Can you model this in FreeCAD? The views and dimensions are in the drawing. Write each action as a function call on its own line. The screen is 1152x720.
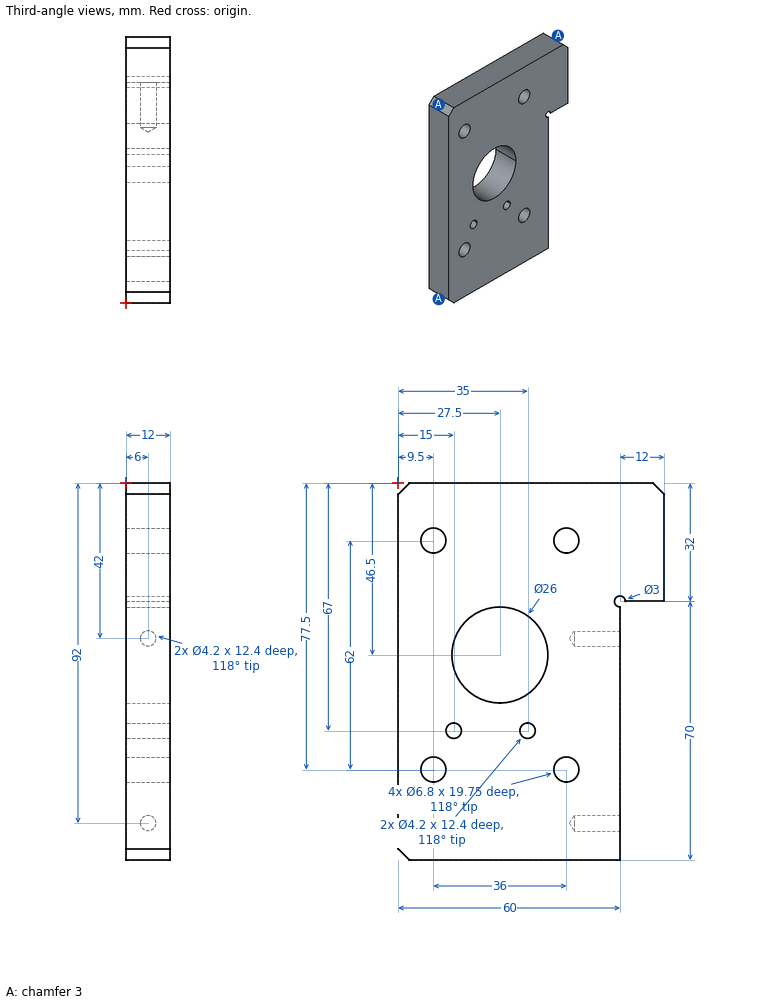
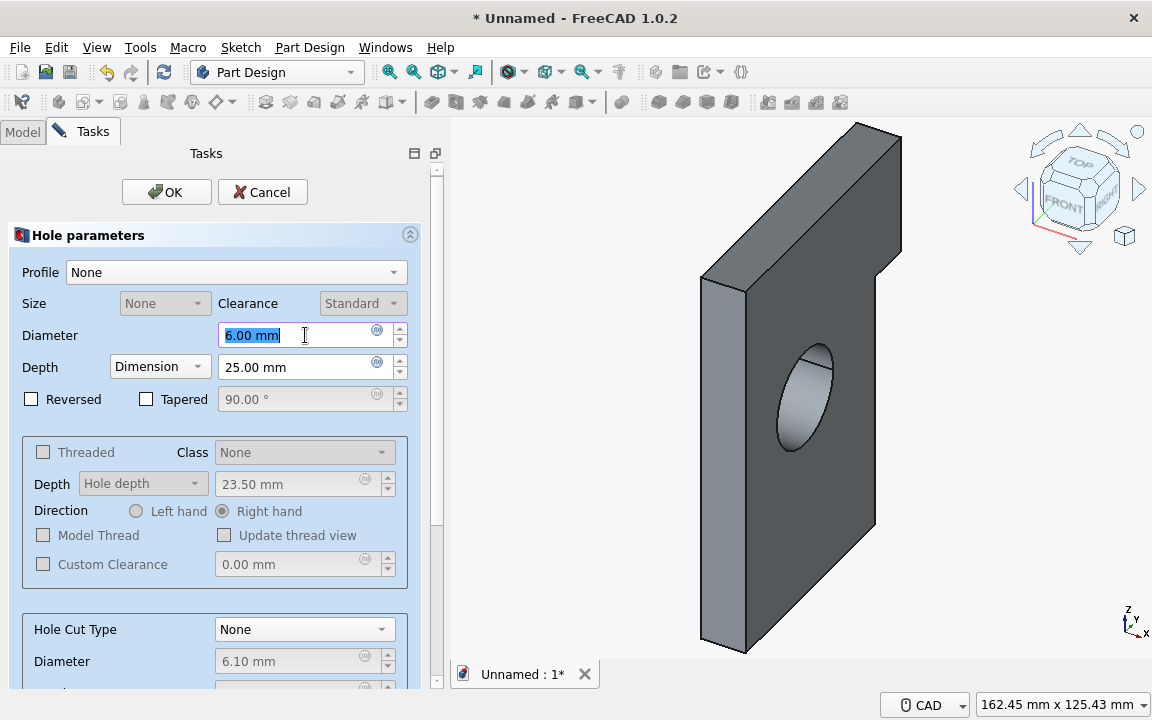
text(6.8)
key(Tab)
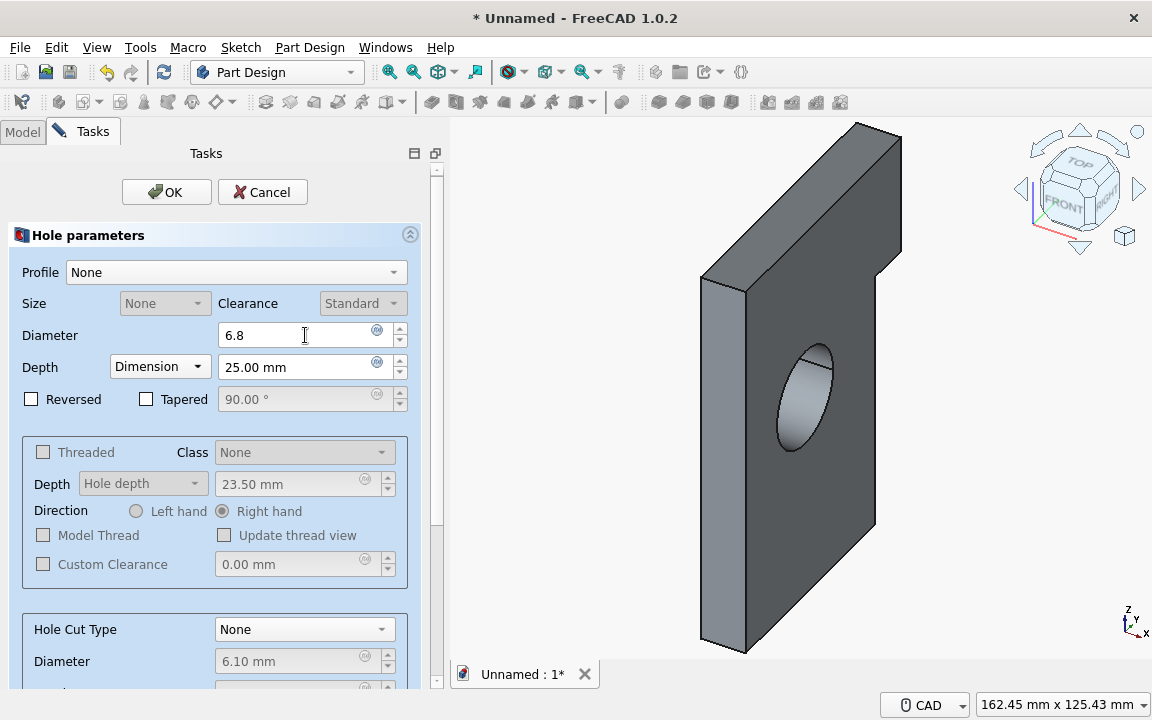
triple_click(305, 367)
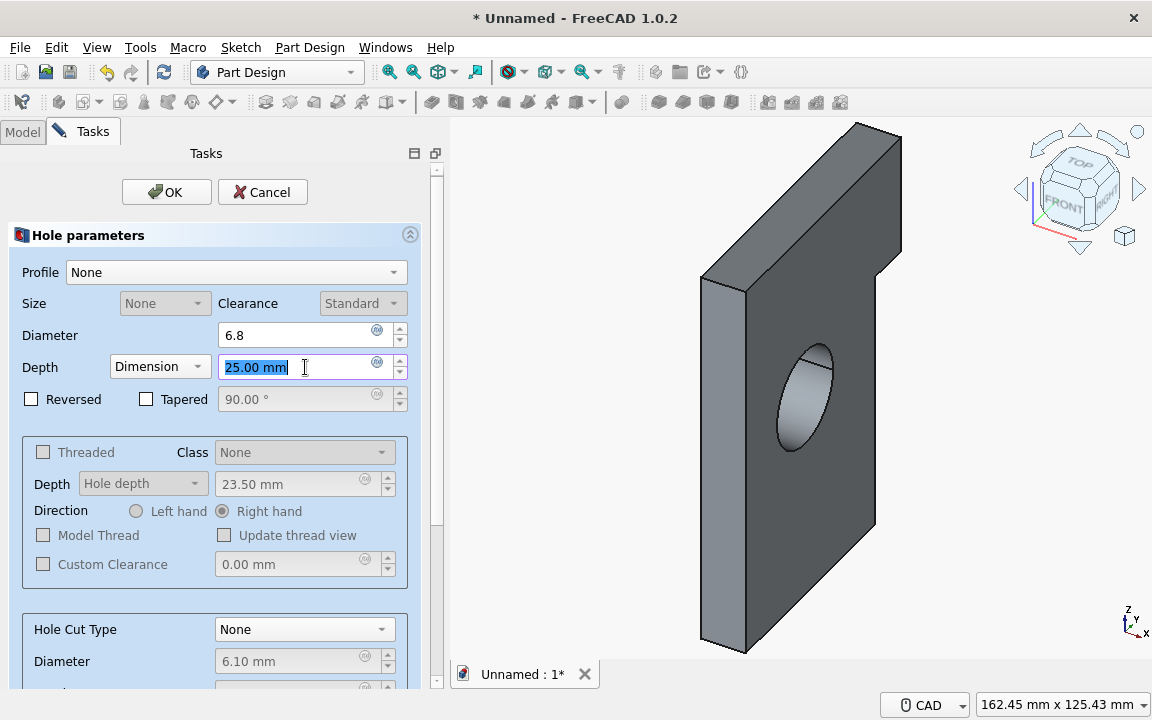
text(19.75)
key(Tab)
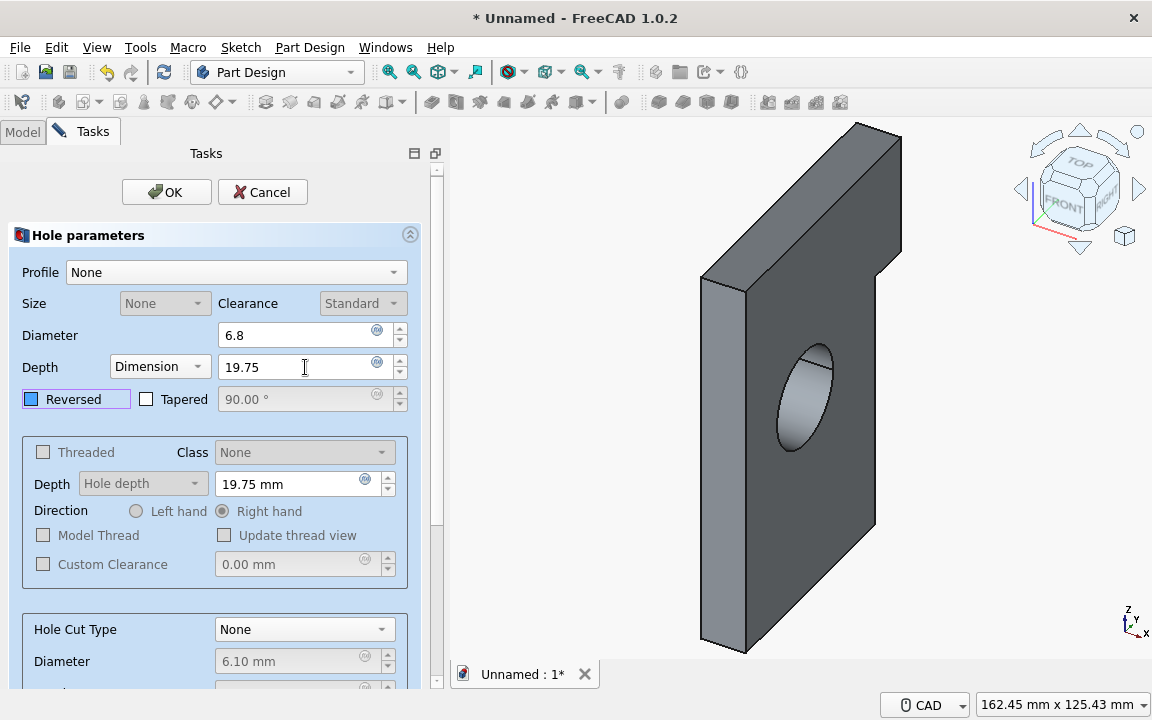
click(30, 399)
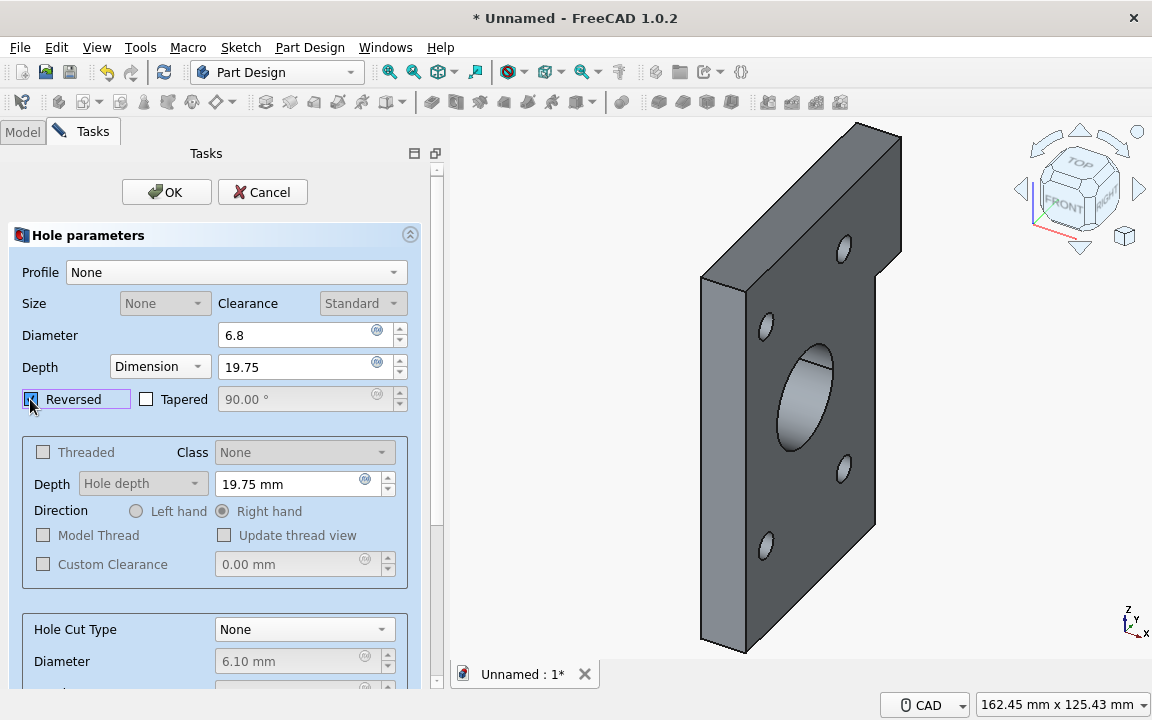
click(167, 192)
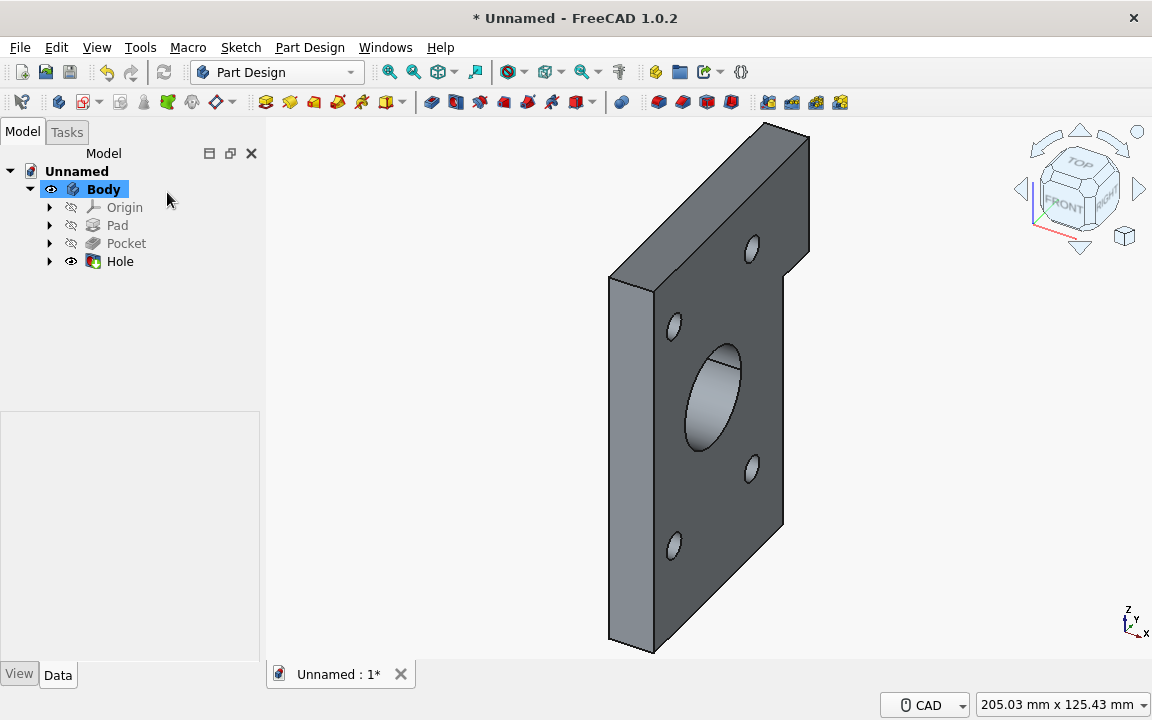
click(709, 520)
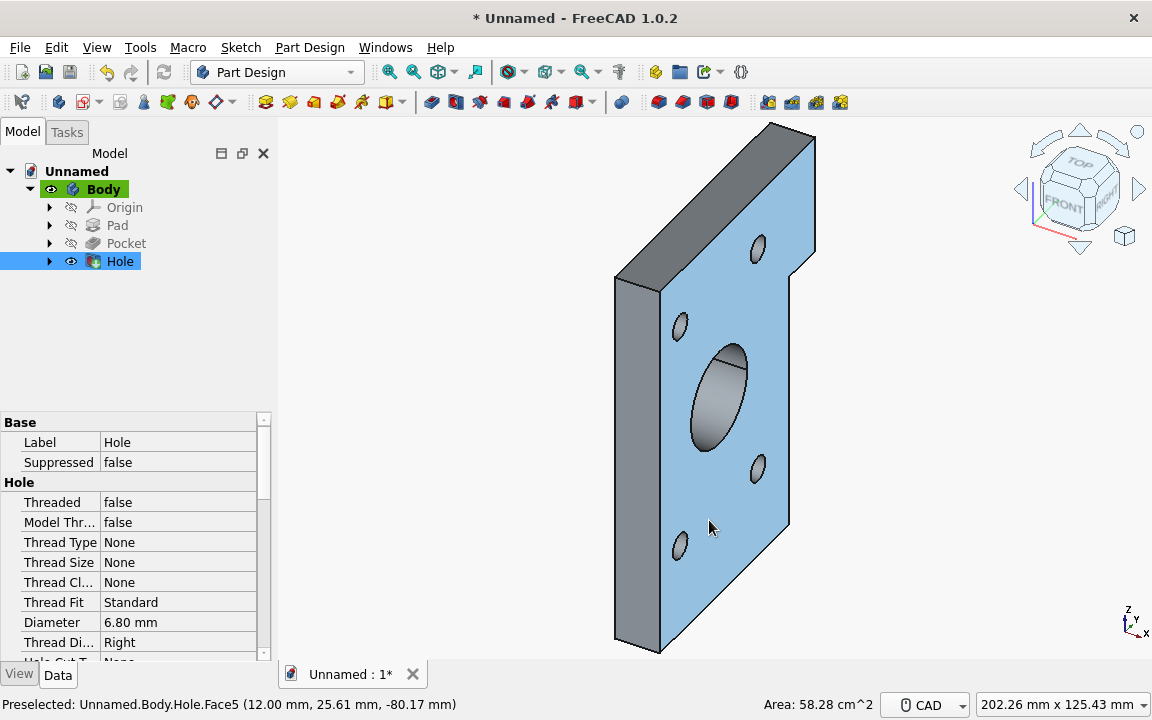
click(84, 102)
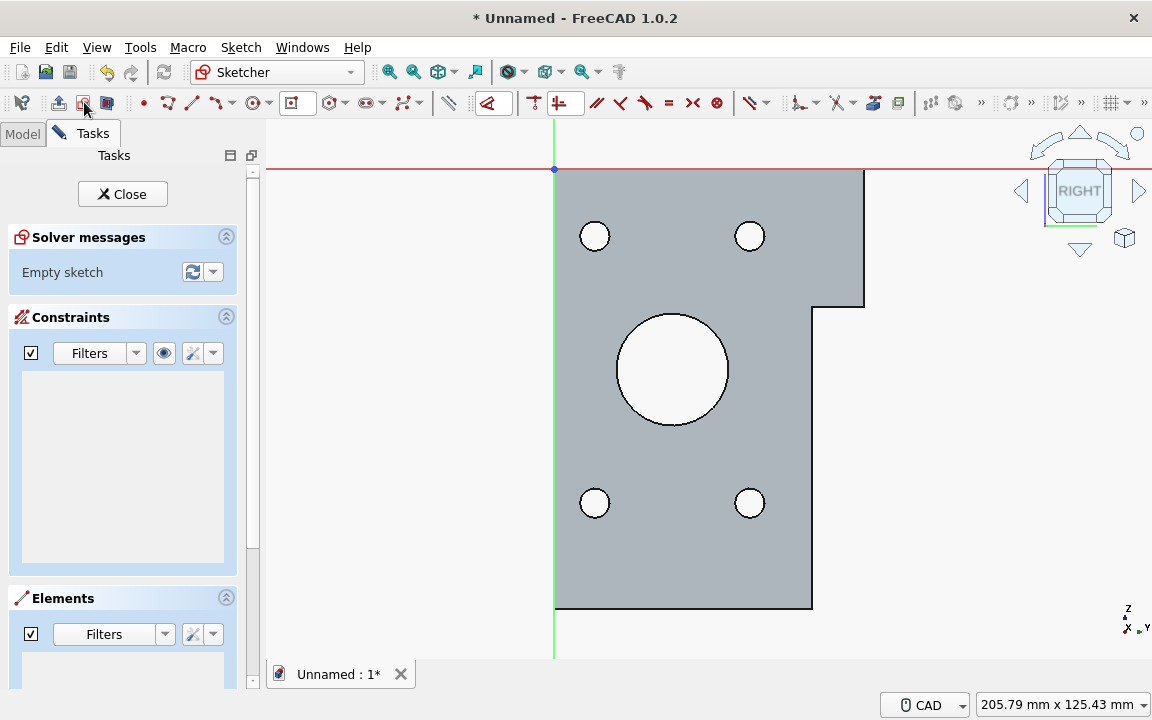
scroll(667, 475, up, 8)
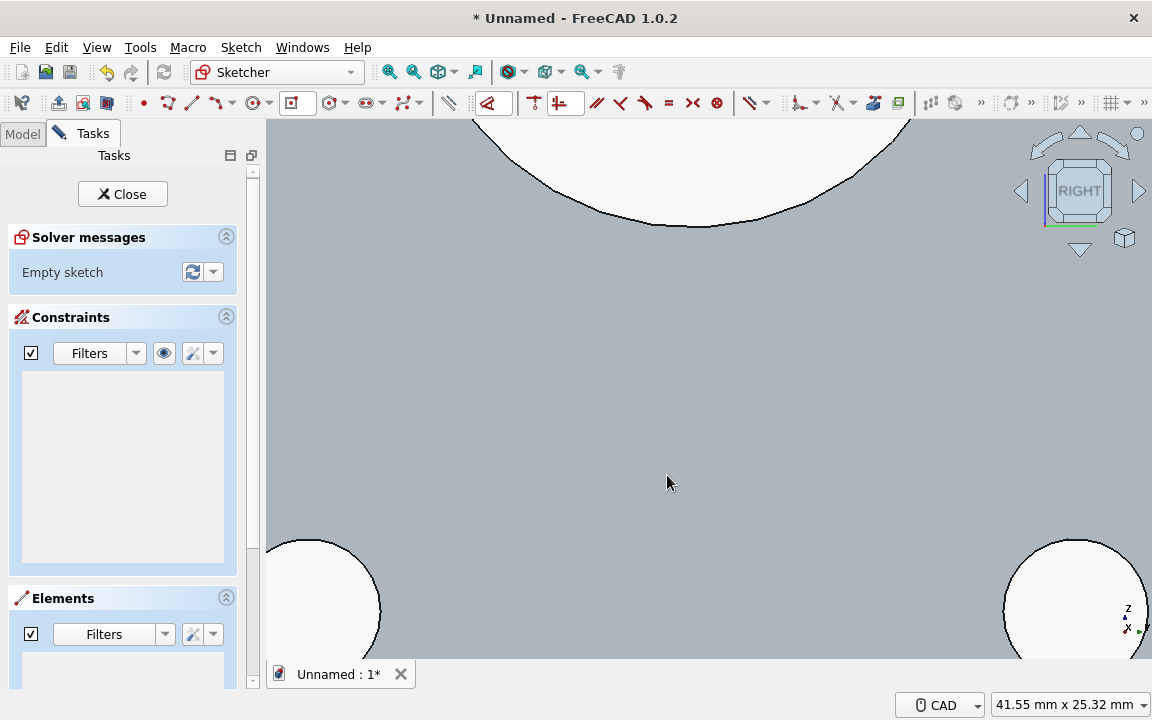
click(254, 104)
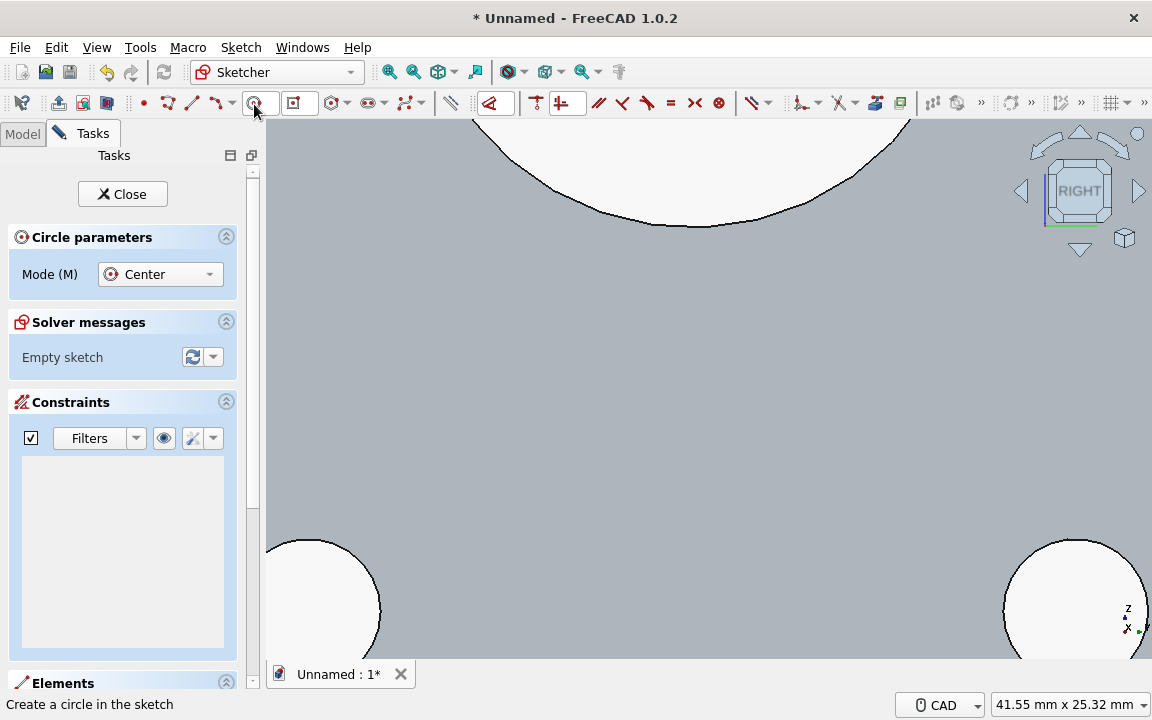
click(852, 388)
move(884, 356)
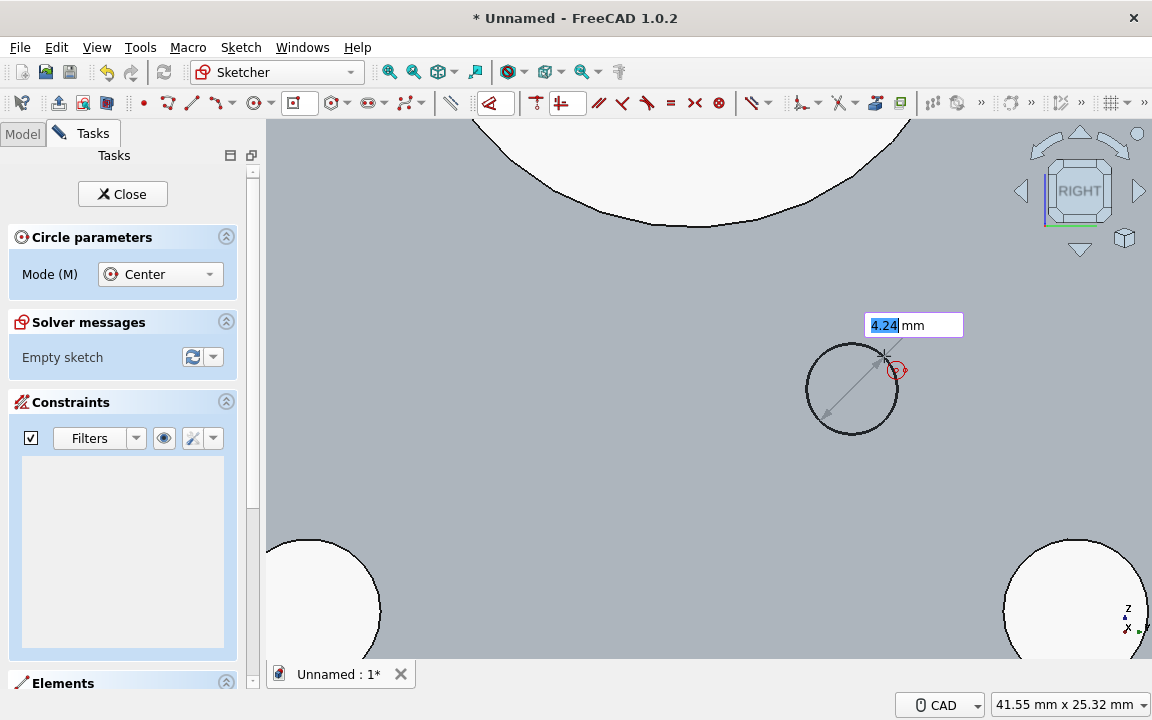
text(4.2)
key(Return)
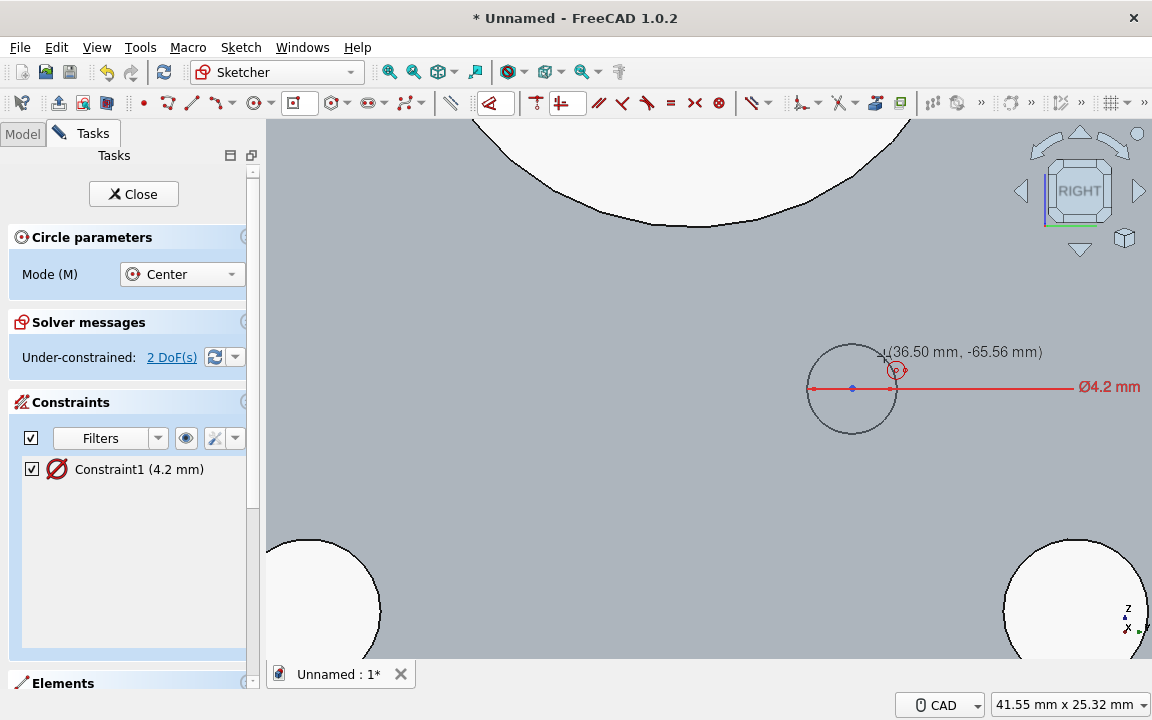
click(425, 388)
move(457, 356)